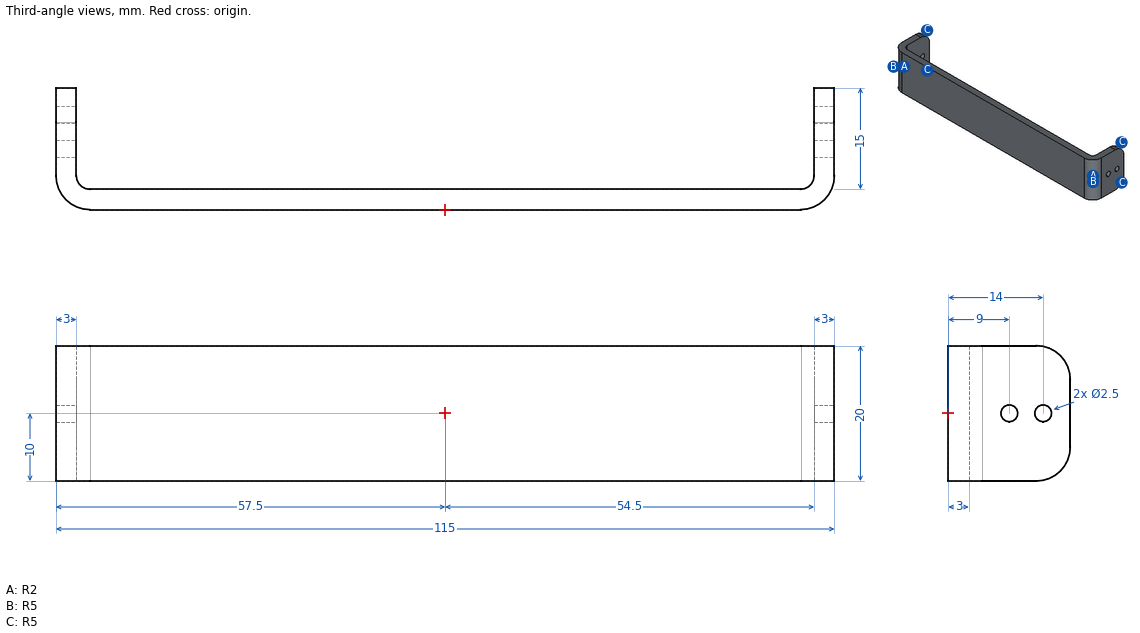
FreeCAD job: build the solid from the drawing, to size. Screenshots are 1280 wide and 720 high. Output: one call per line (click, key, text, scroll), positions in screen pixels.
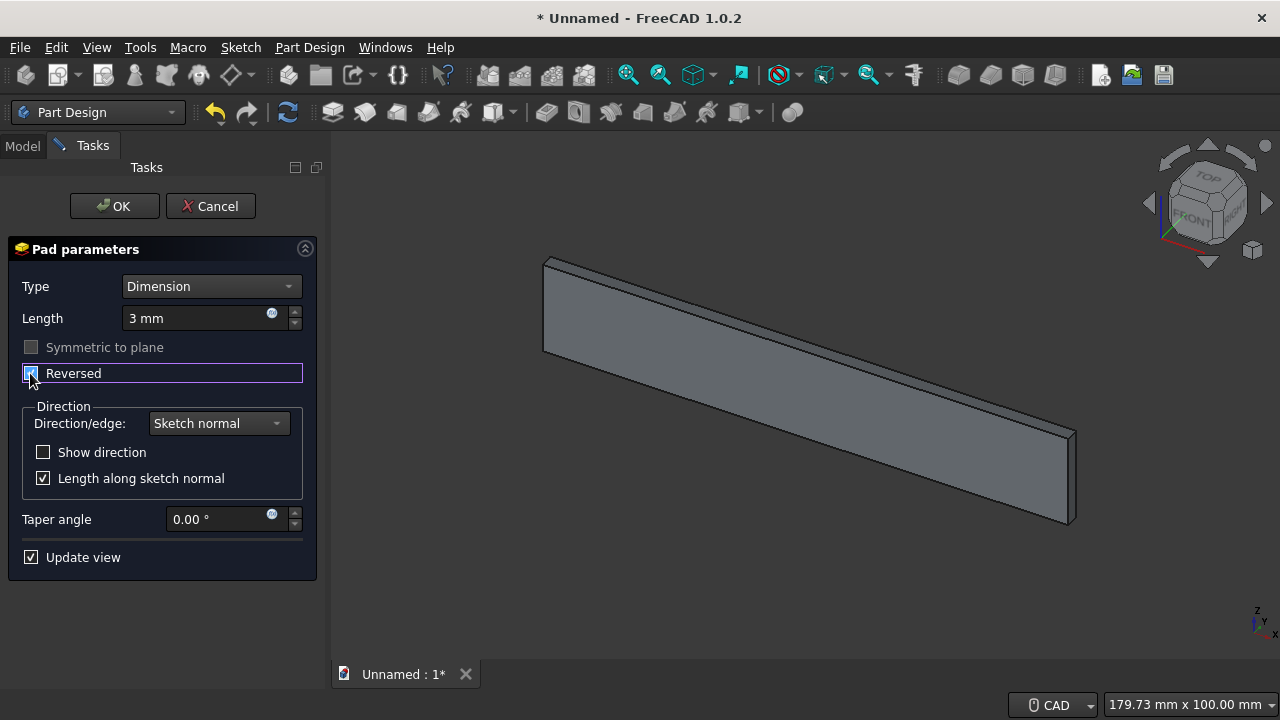
click(115, 206)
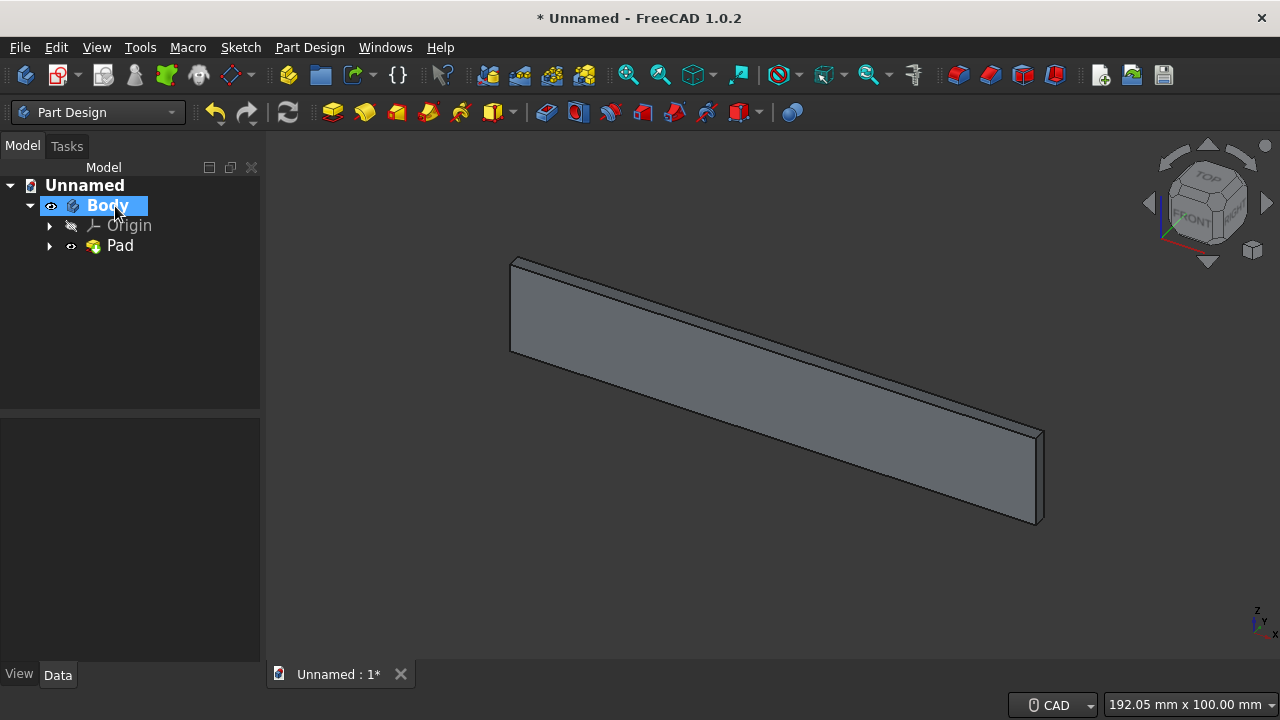
key(4)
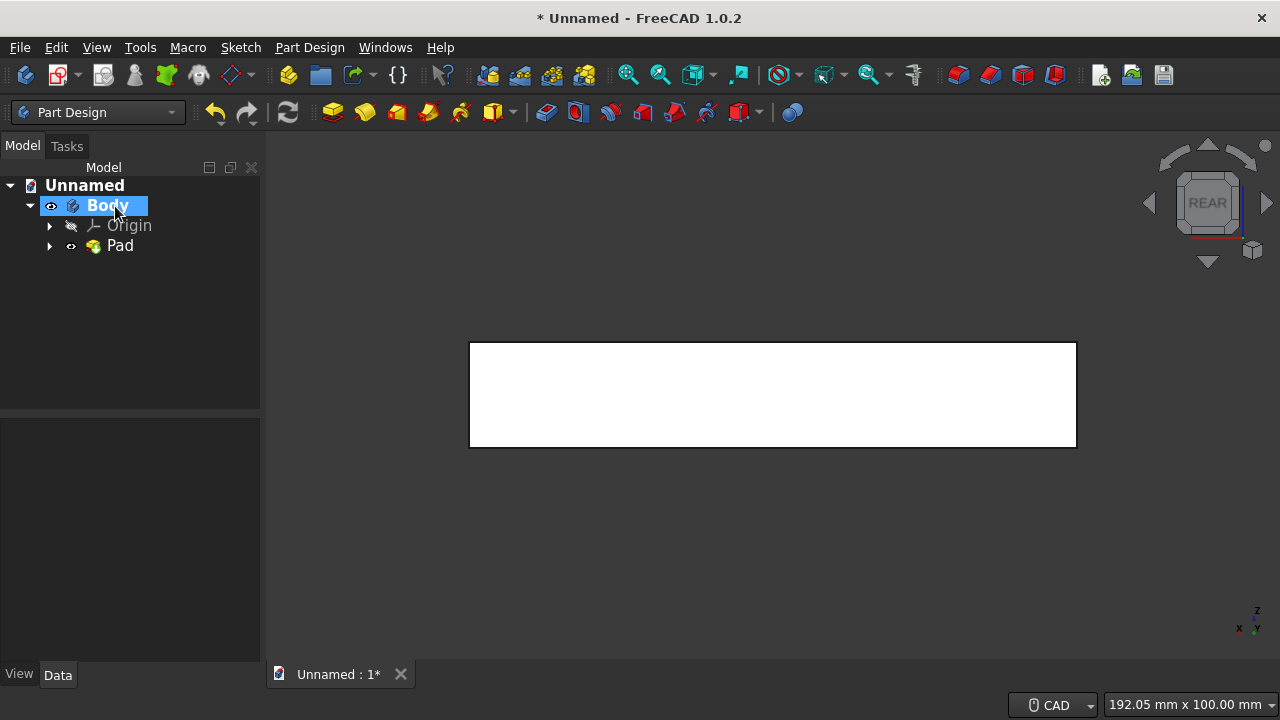
click(600, 394)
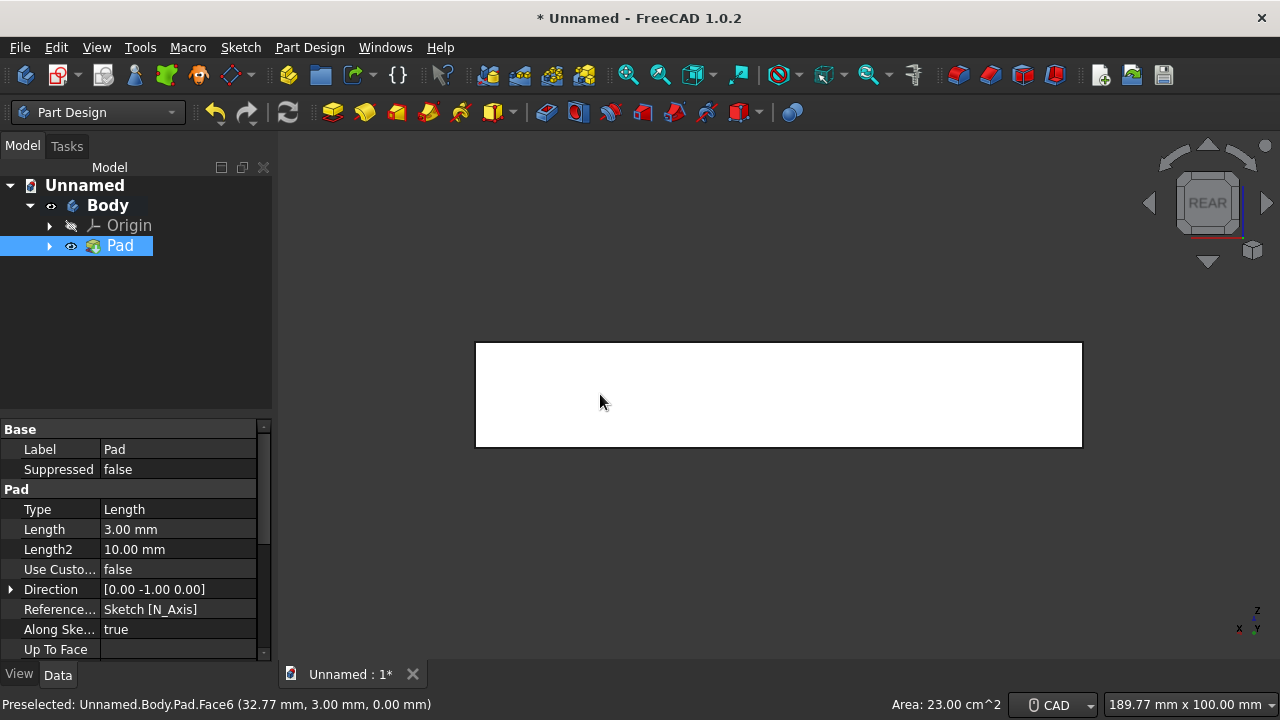
click(58, 76)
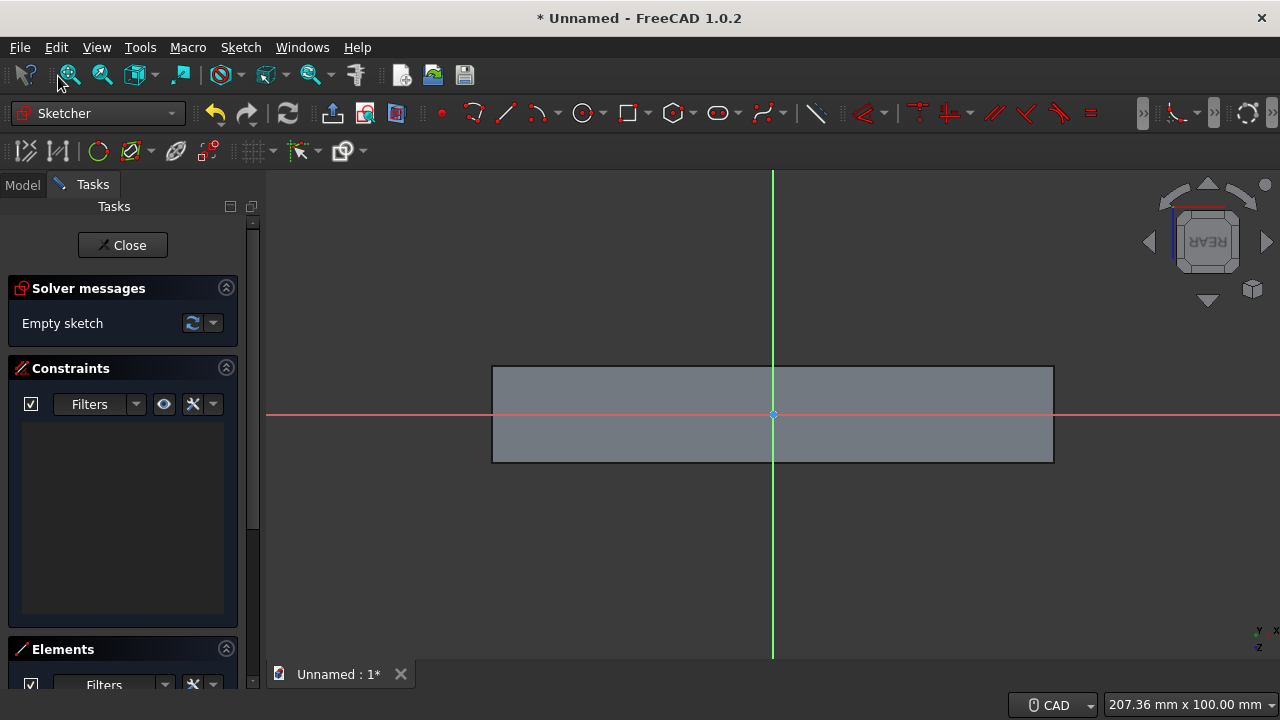
key(g)
key(r)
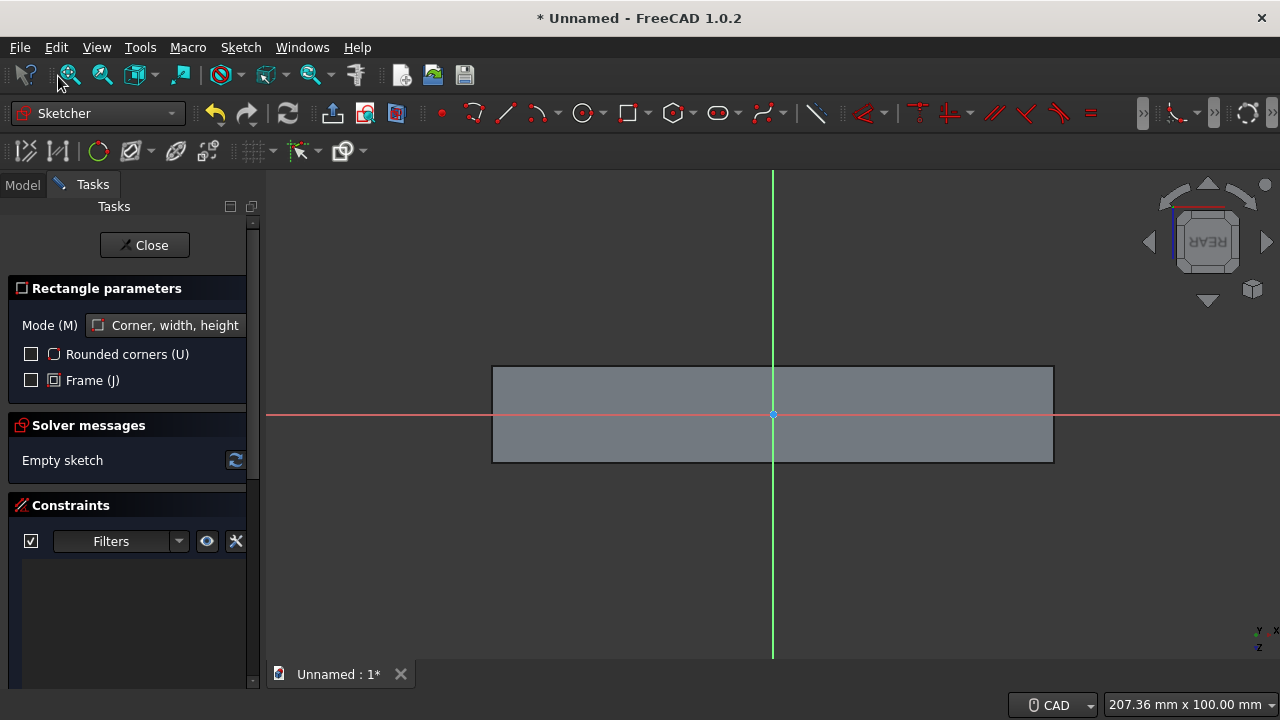
click(492, 366)
move(506, 463)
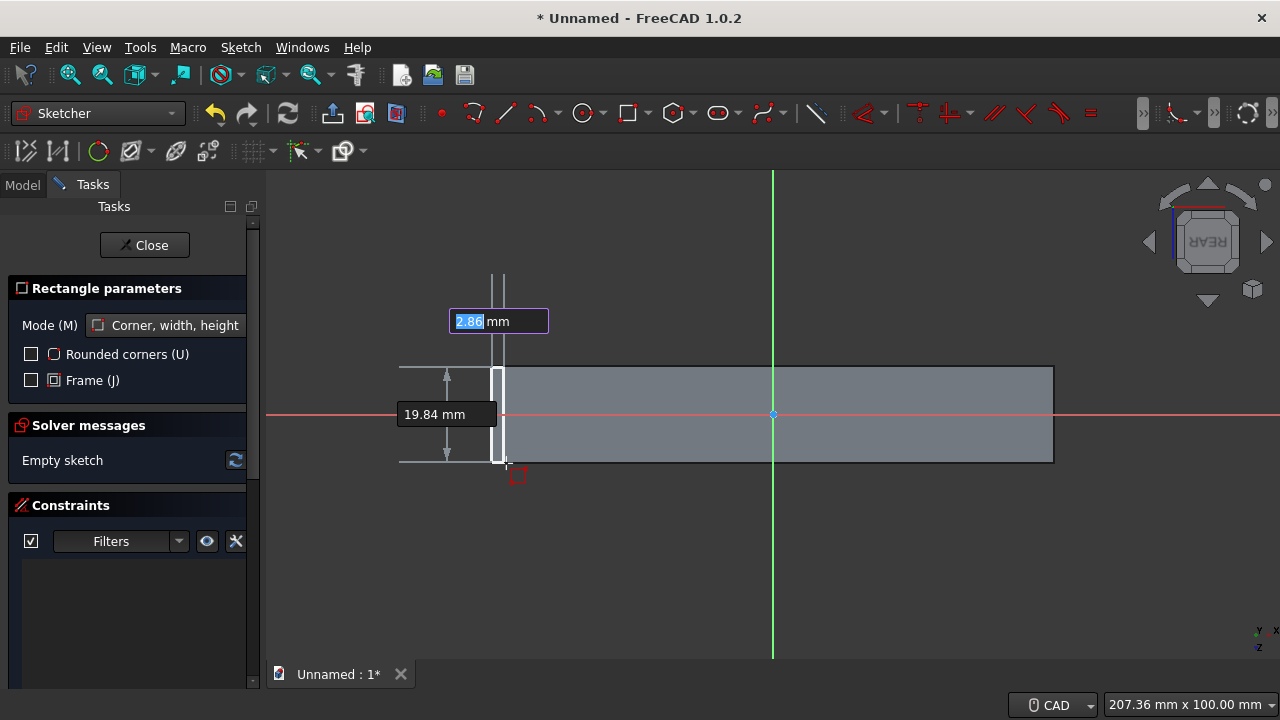
text(3)
key(Tab)
text(20)
key(Return)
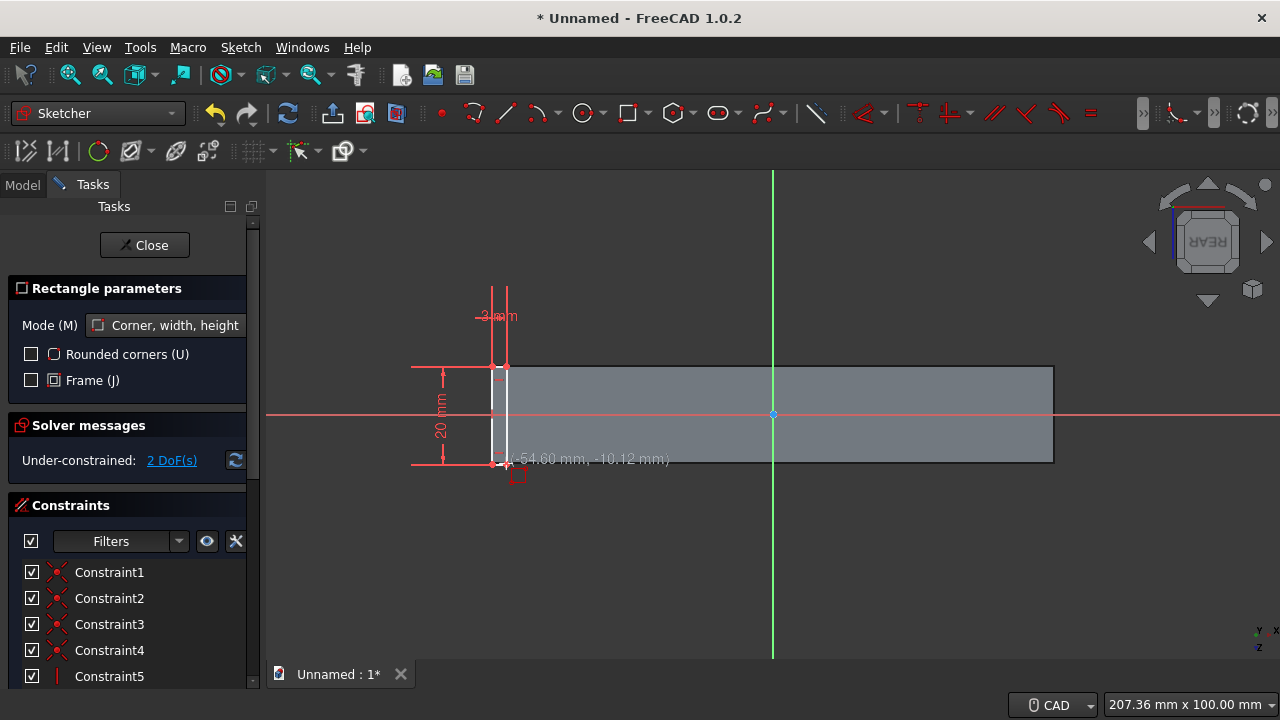
click(1040, 366)
move(1054, 463)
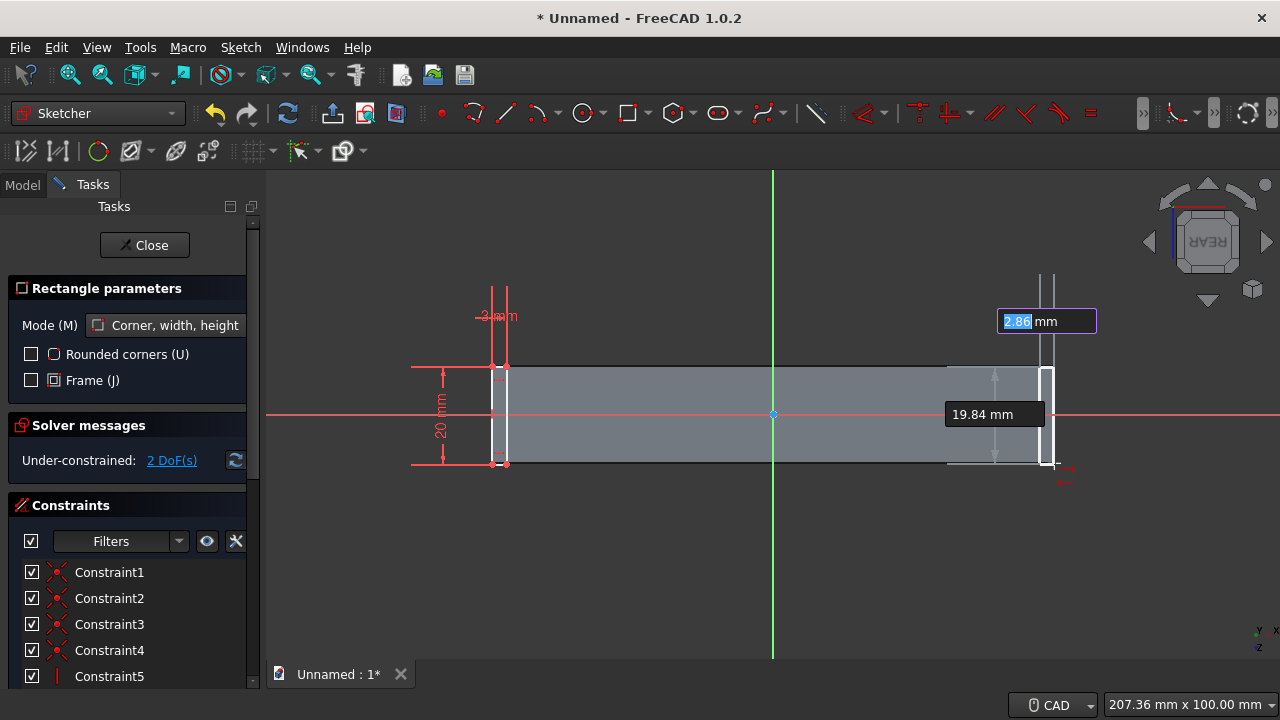
text(3)
key(Tab)
text(20)
key(Return)
key(Escape)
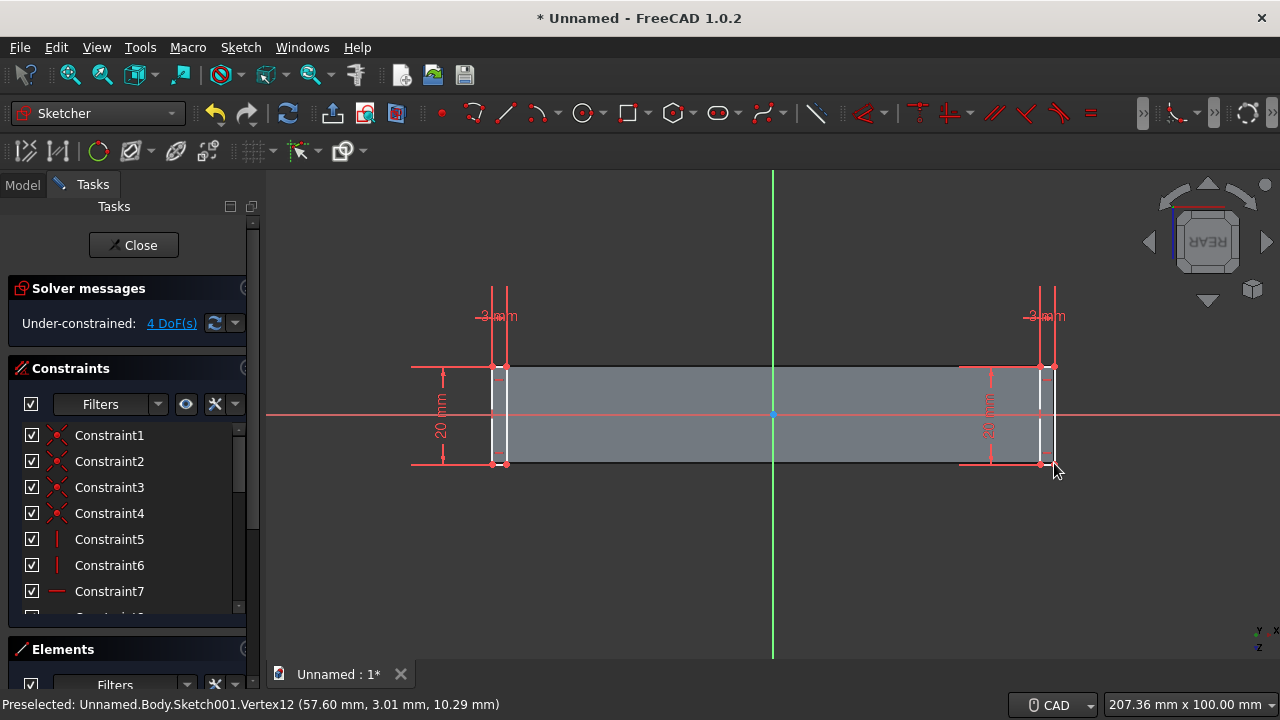
click(492, 367)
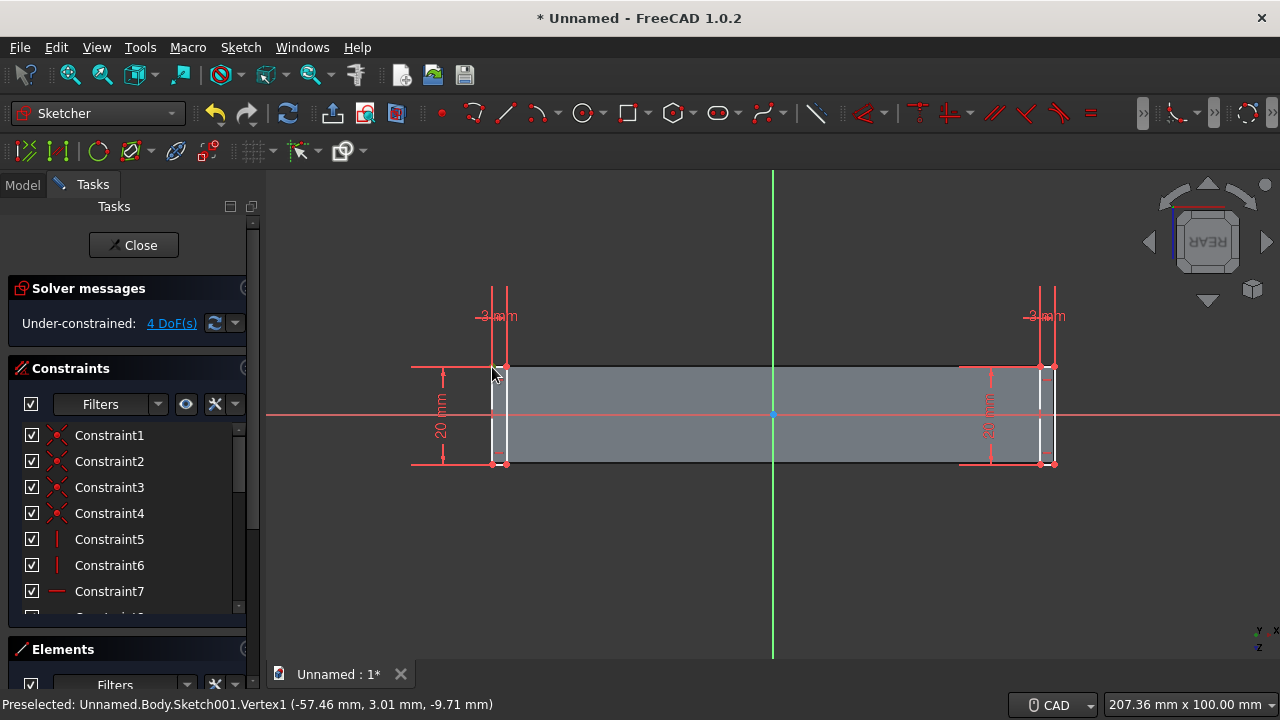
click(886, 114)